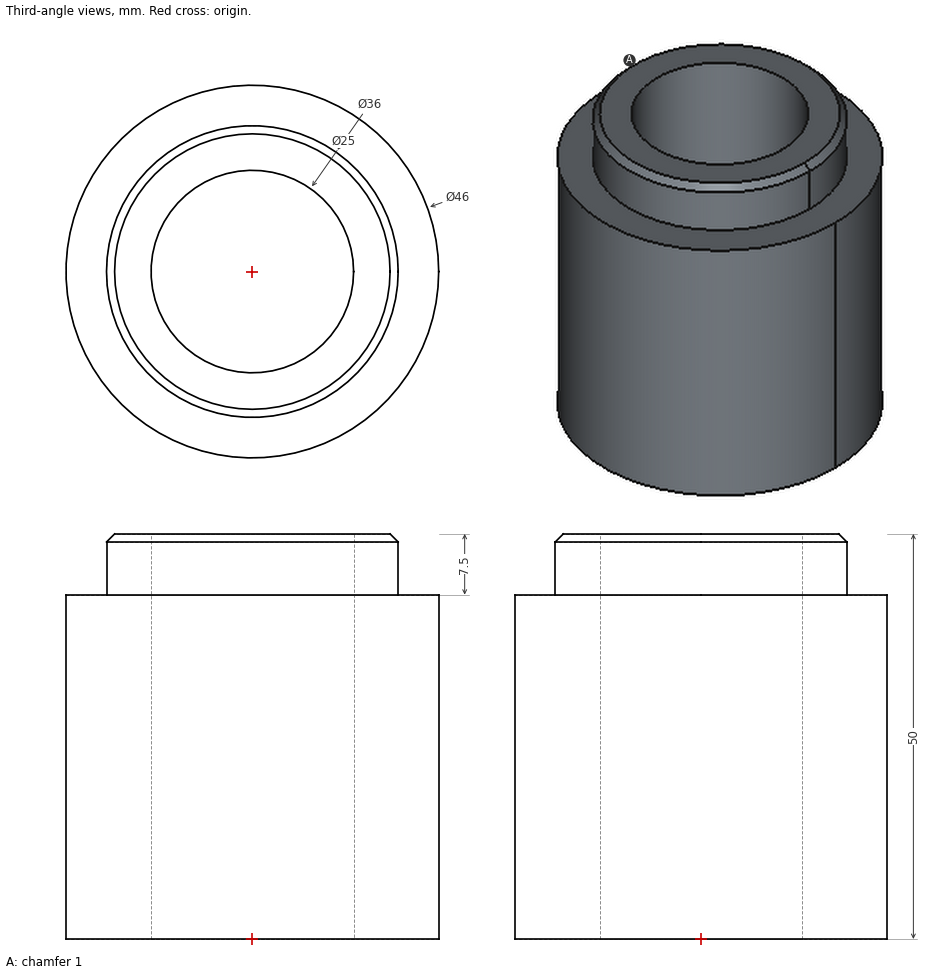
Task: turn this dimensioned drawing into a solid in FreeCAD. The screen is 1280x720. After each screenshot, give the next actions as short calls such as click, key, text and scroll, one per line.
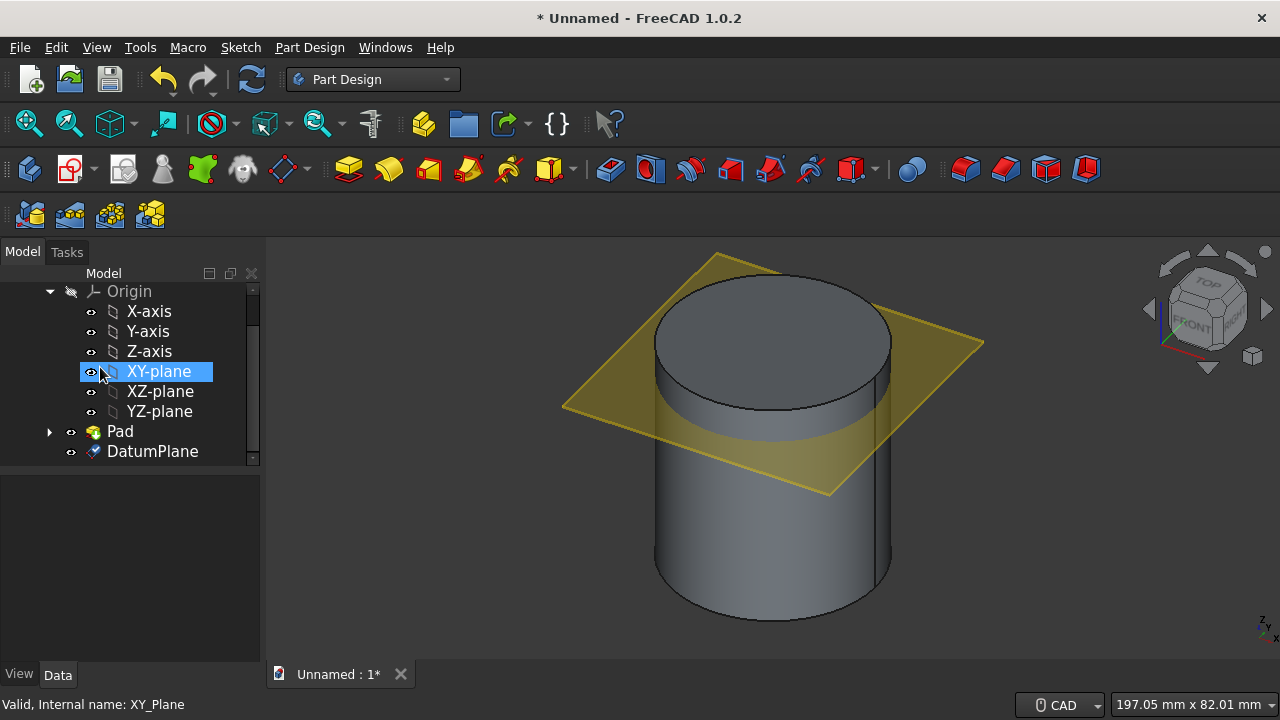
click(116, 452)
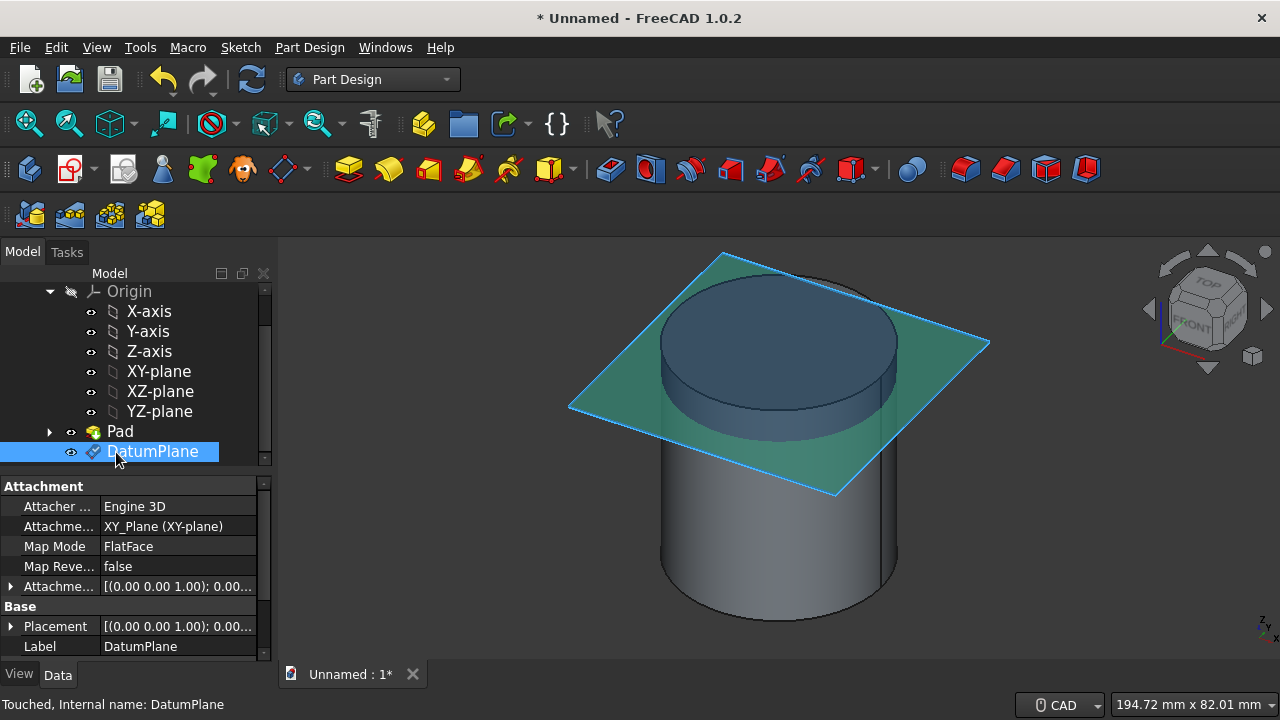
click(70, 170)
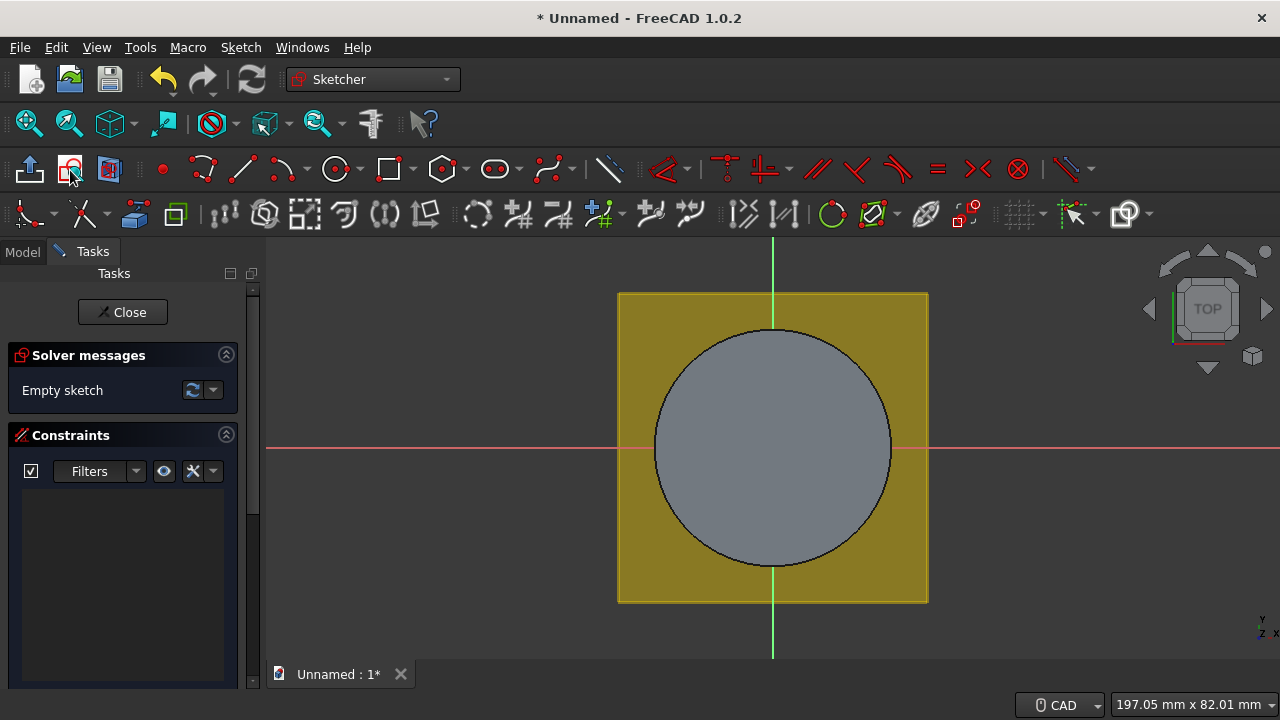
click(110, 170)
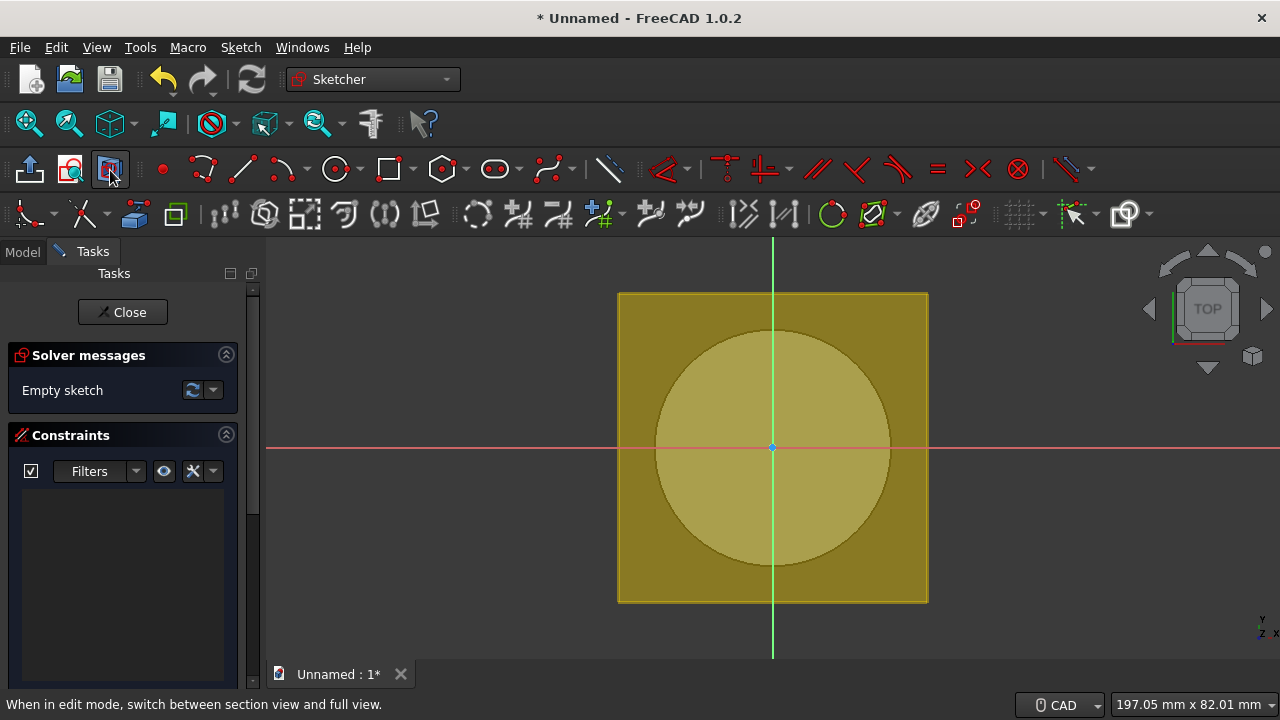
key(g)
key(c)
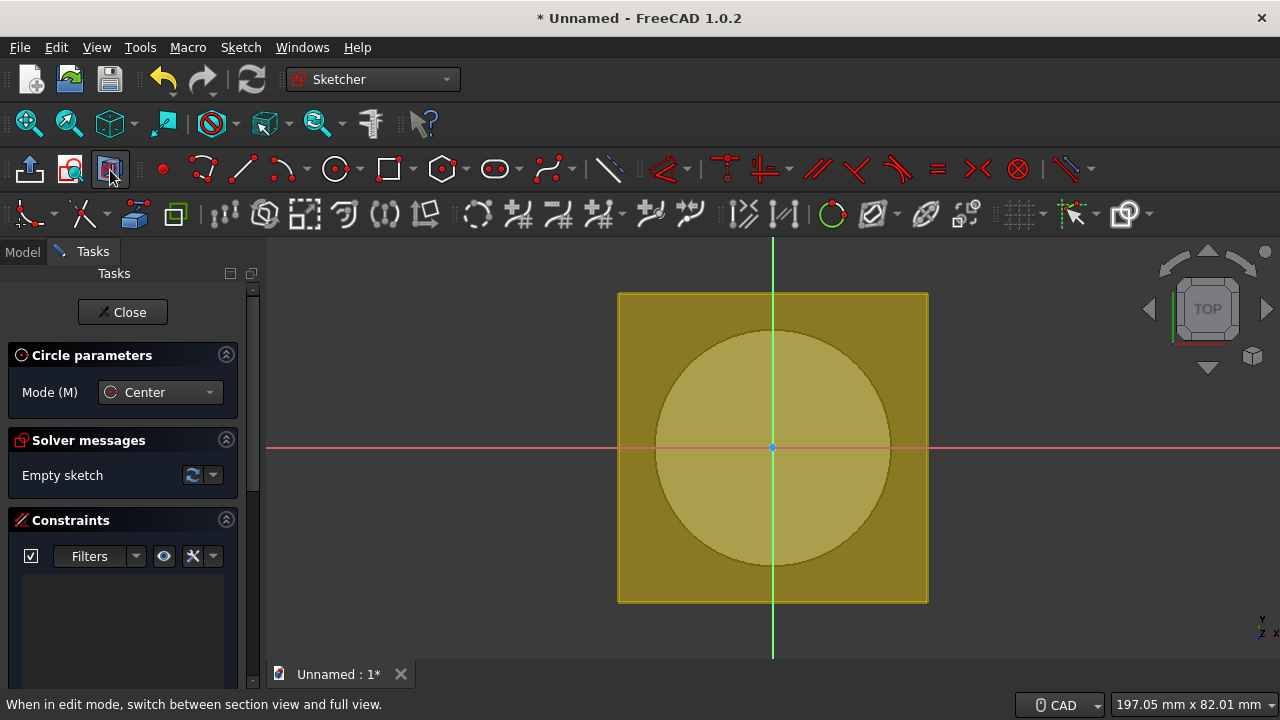
click(773, 448)
move(857, 364)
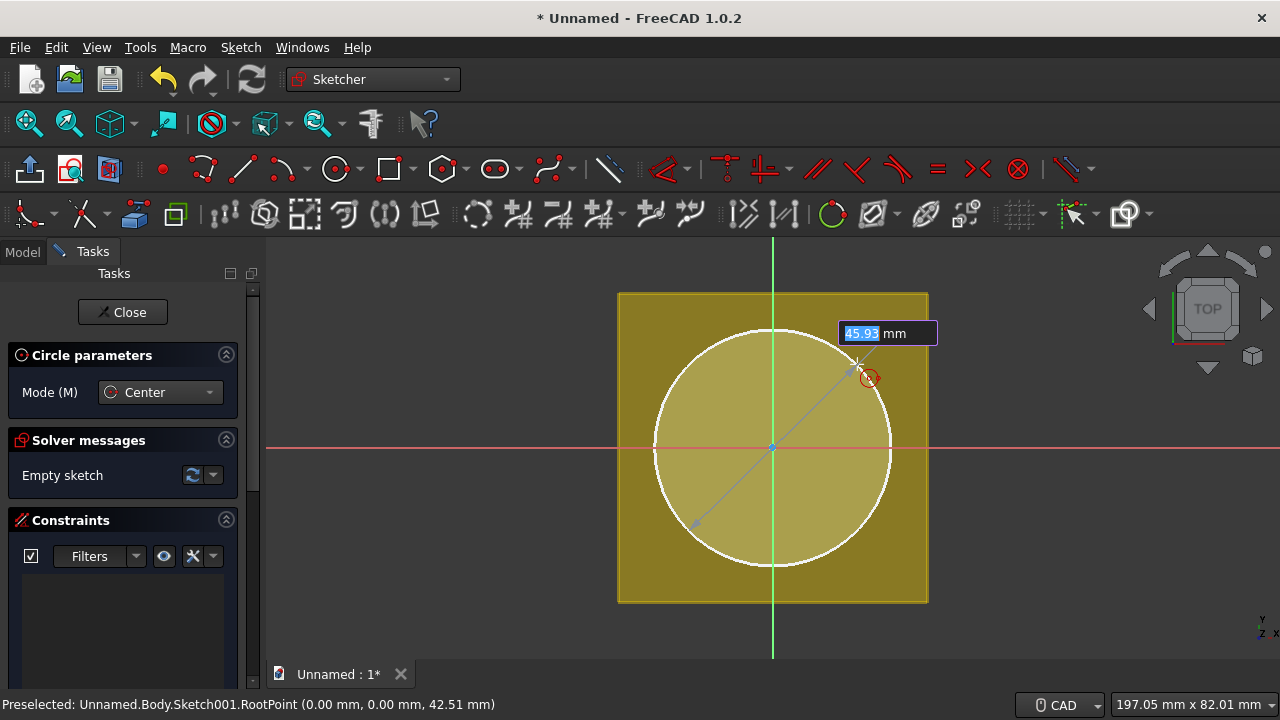
text(46)
key(Return)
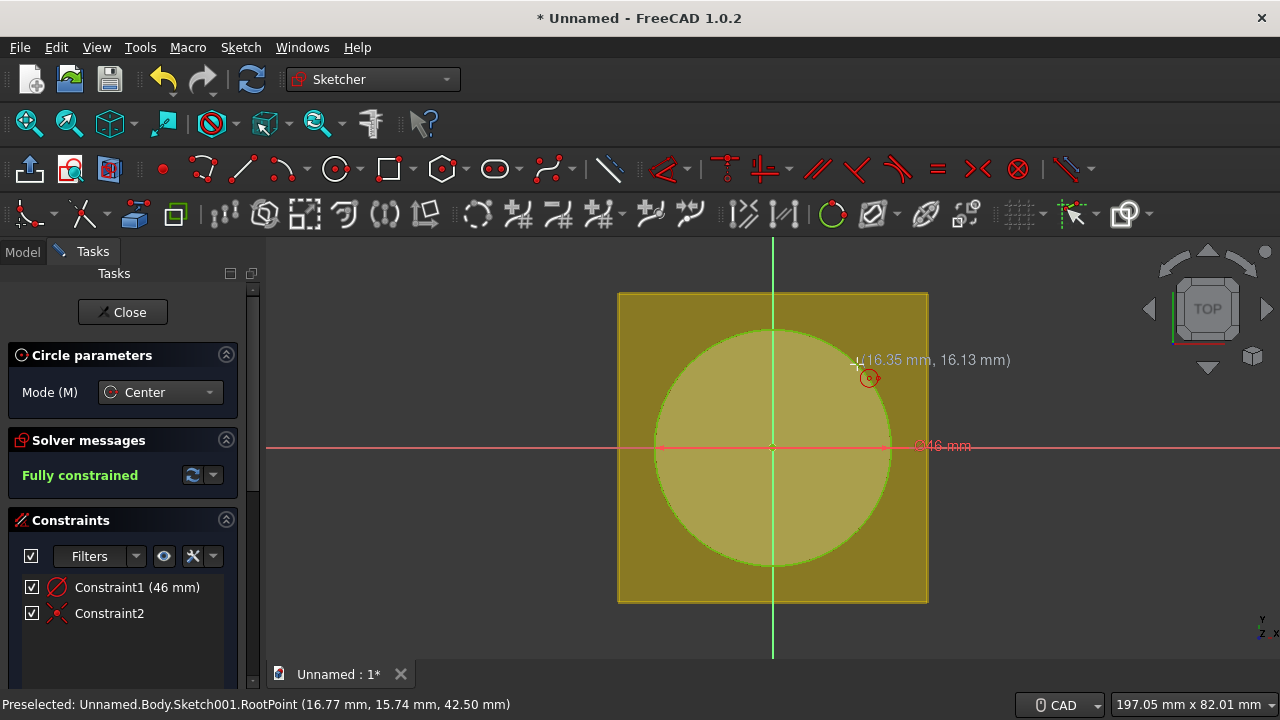
click(773, 448)
move(838, 383)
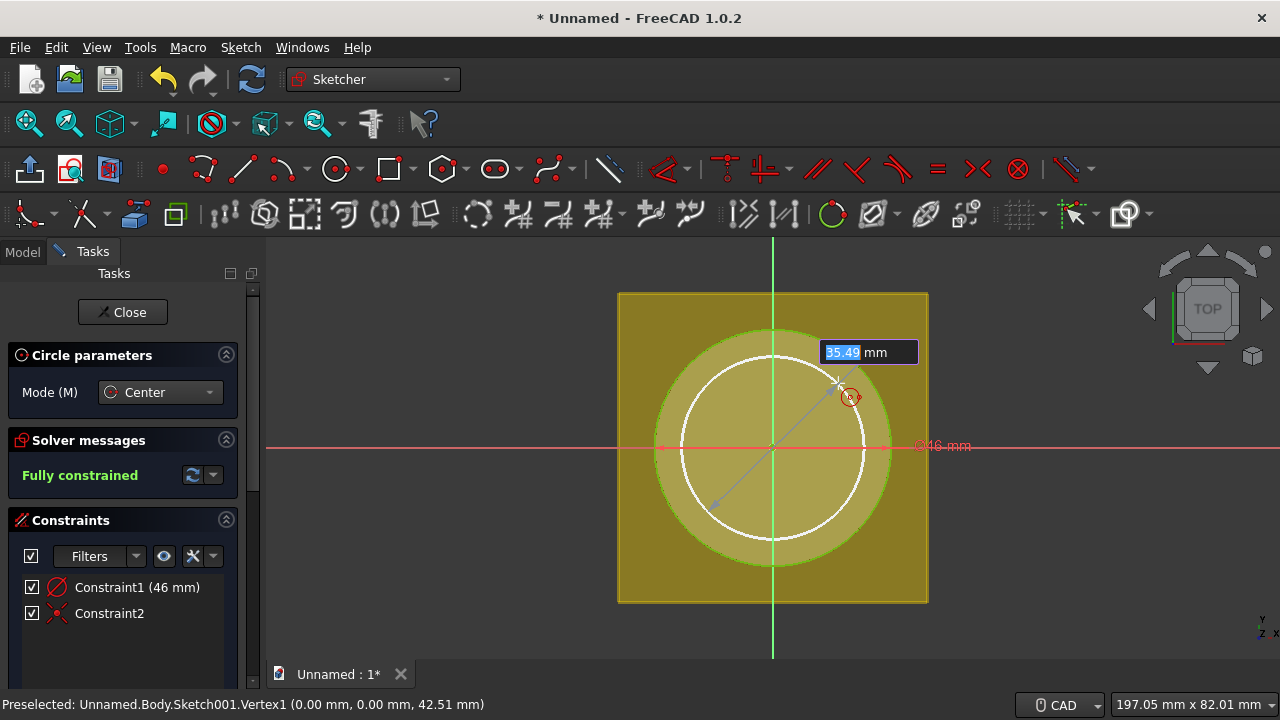
text(36)
key(Return)
key(Escape)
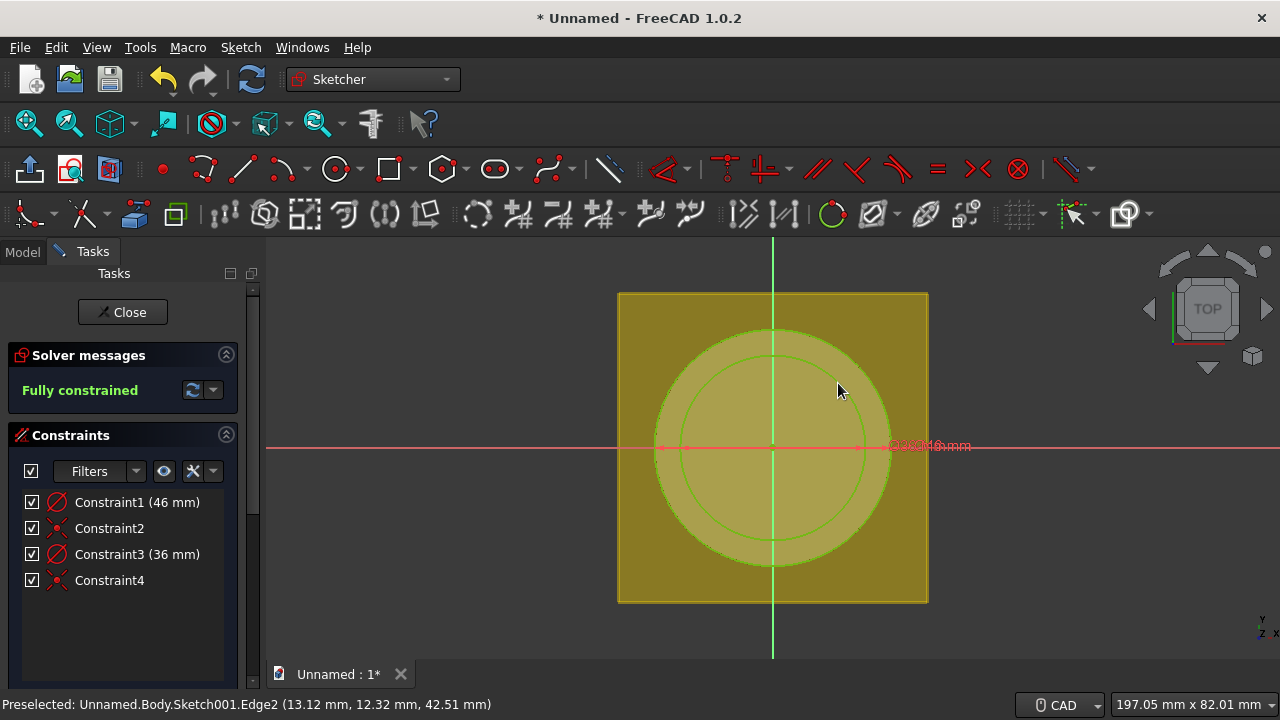
click(123, 312)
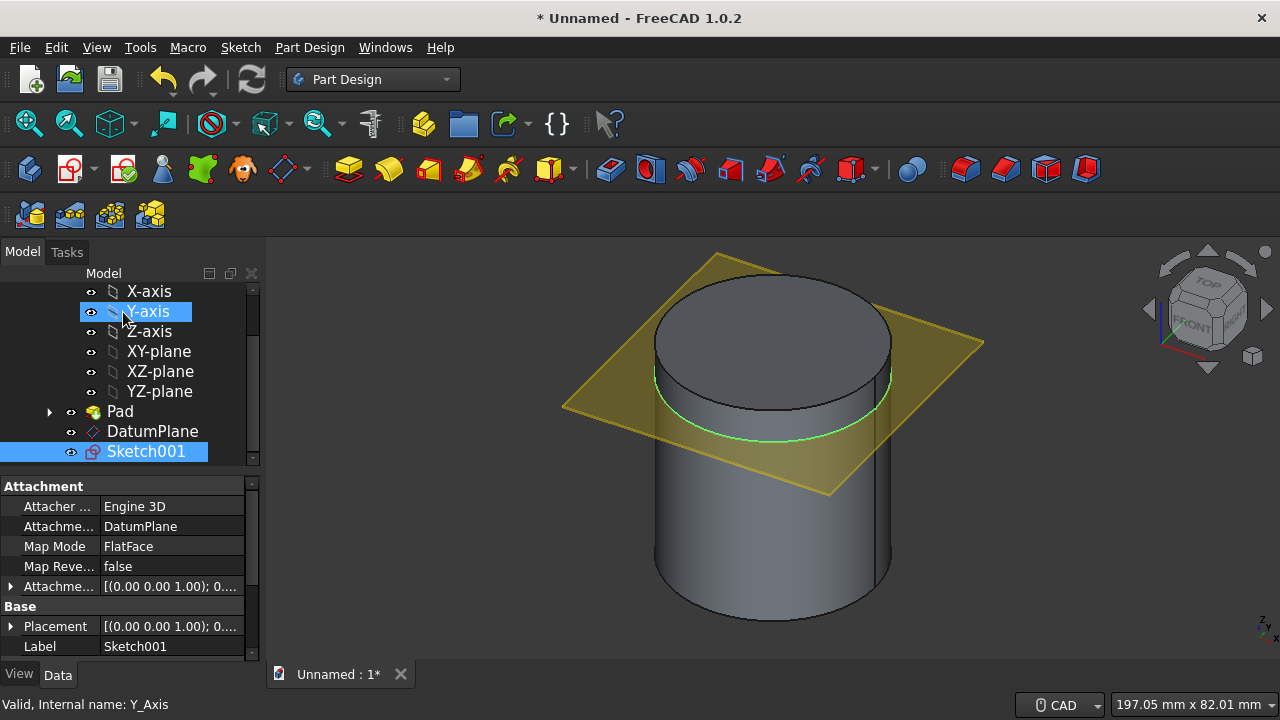
click(612, 170)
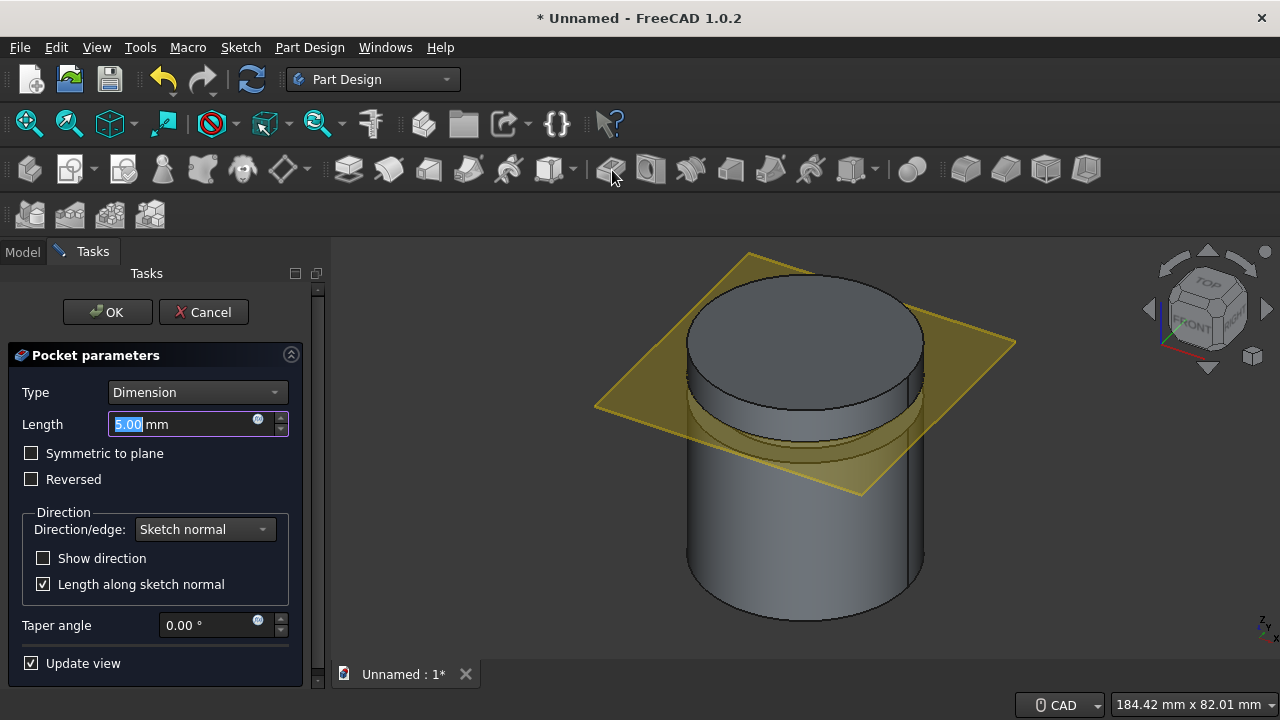
text(7.5)
key(Tab)